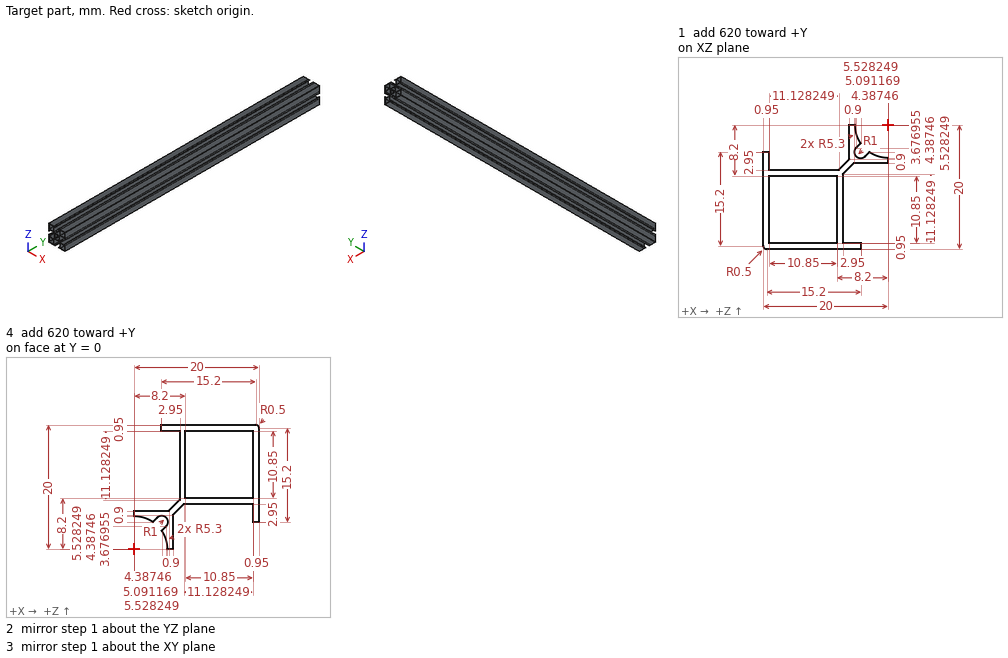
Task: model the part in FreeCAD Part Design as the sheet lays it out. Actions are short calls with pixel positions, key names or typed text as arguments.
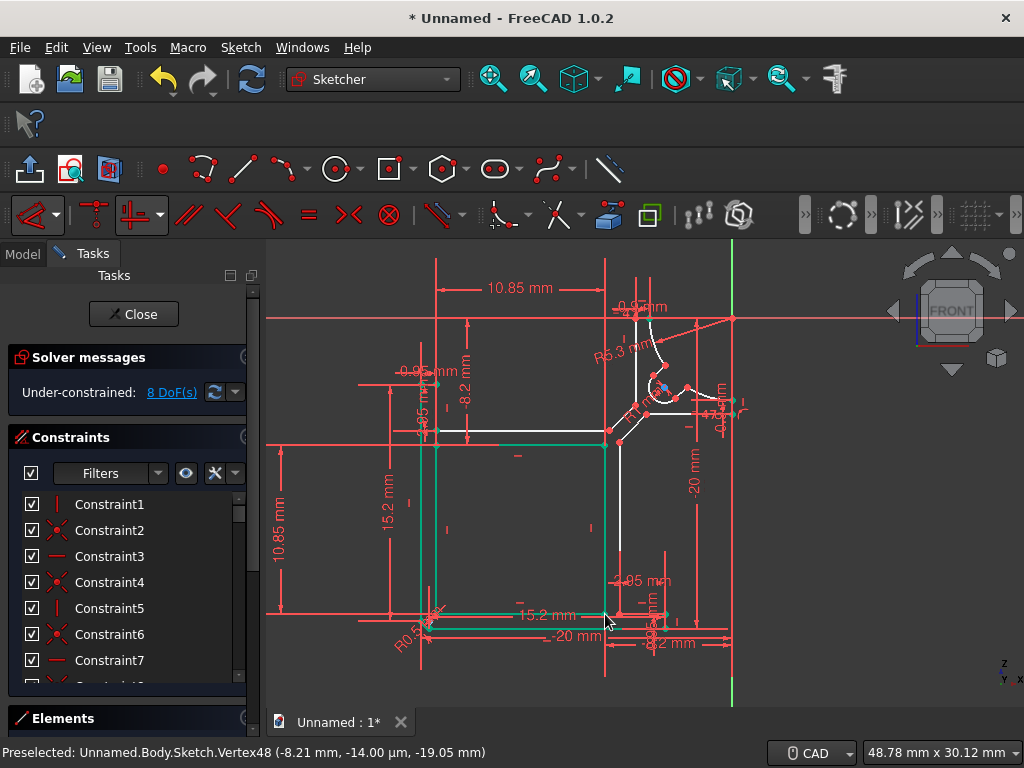
click(636, 379)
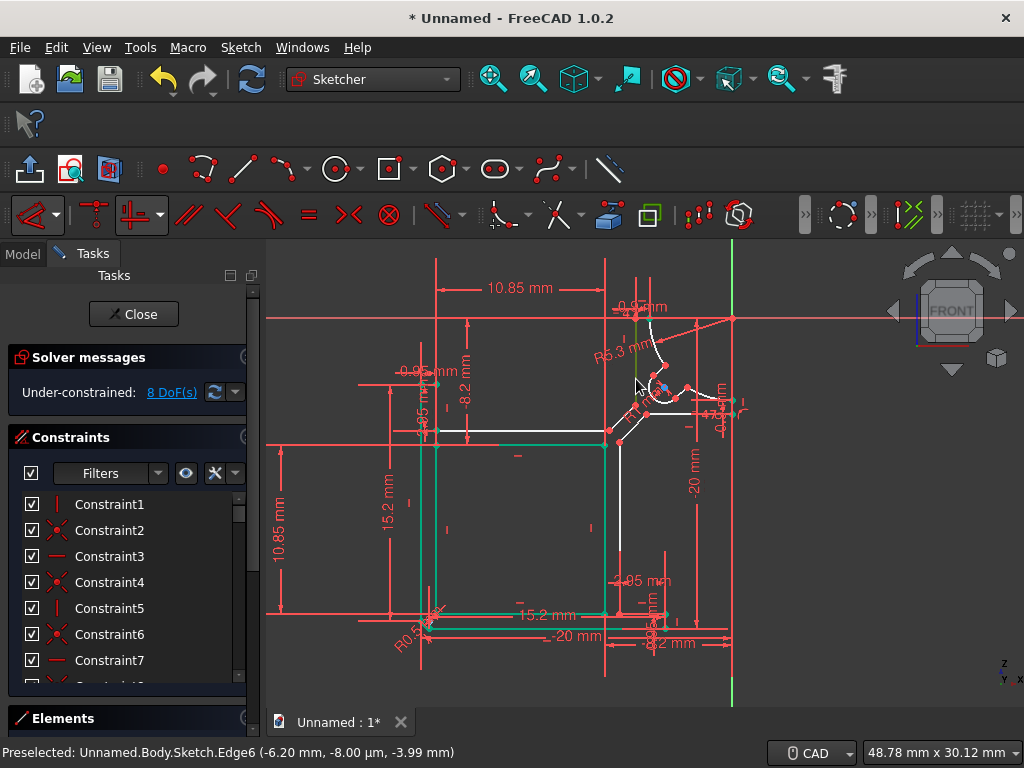
click(58, 216)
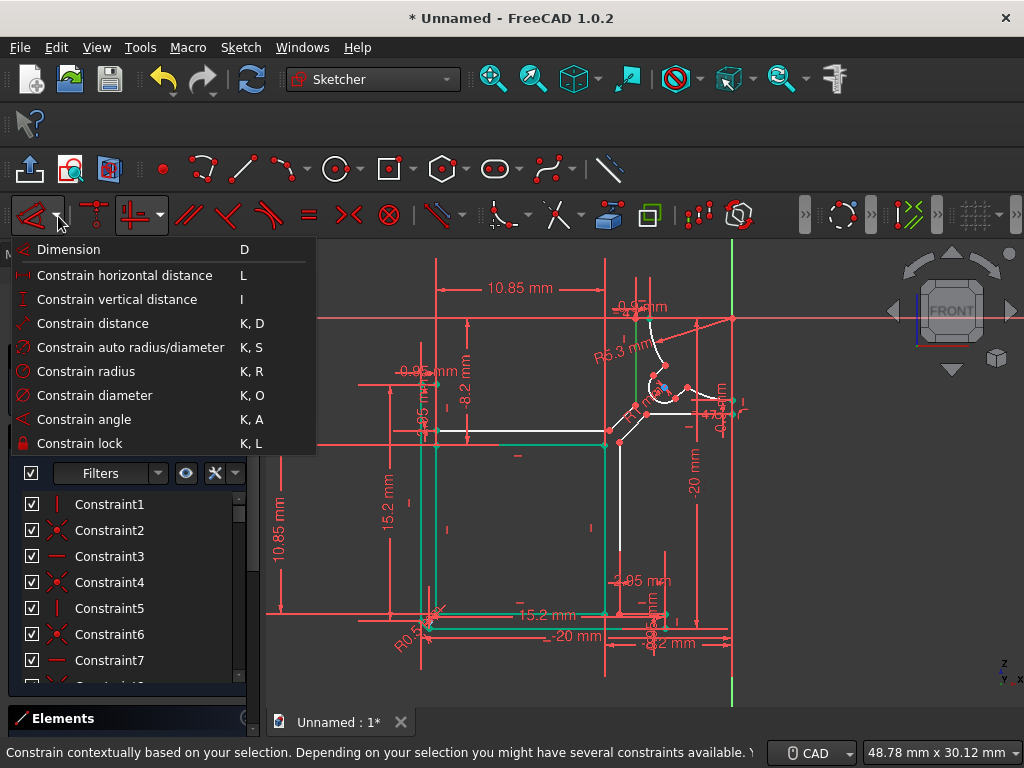
click(164, 299)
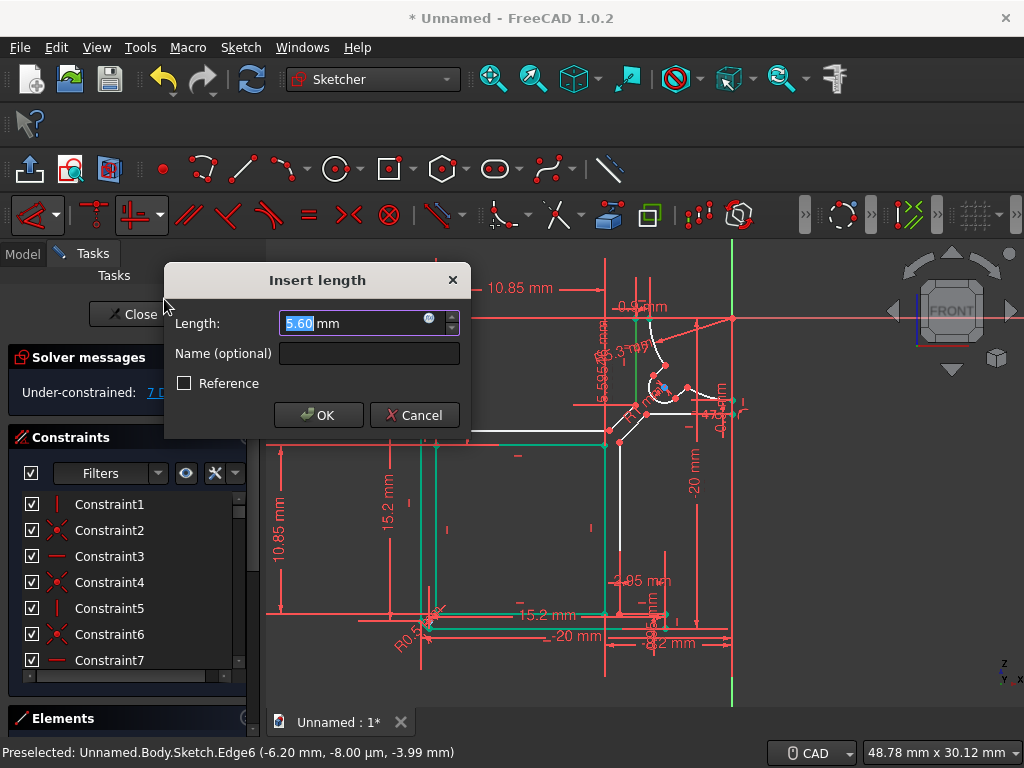
text(5.528249)
key(Return)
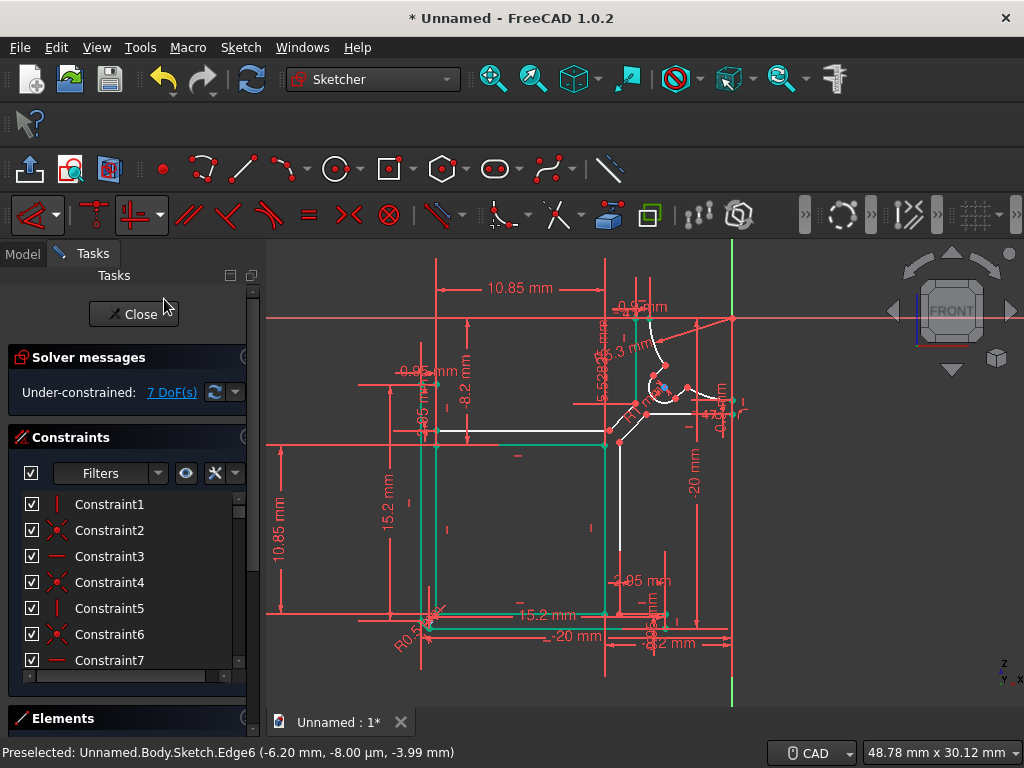
click(672, 414)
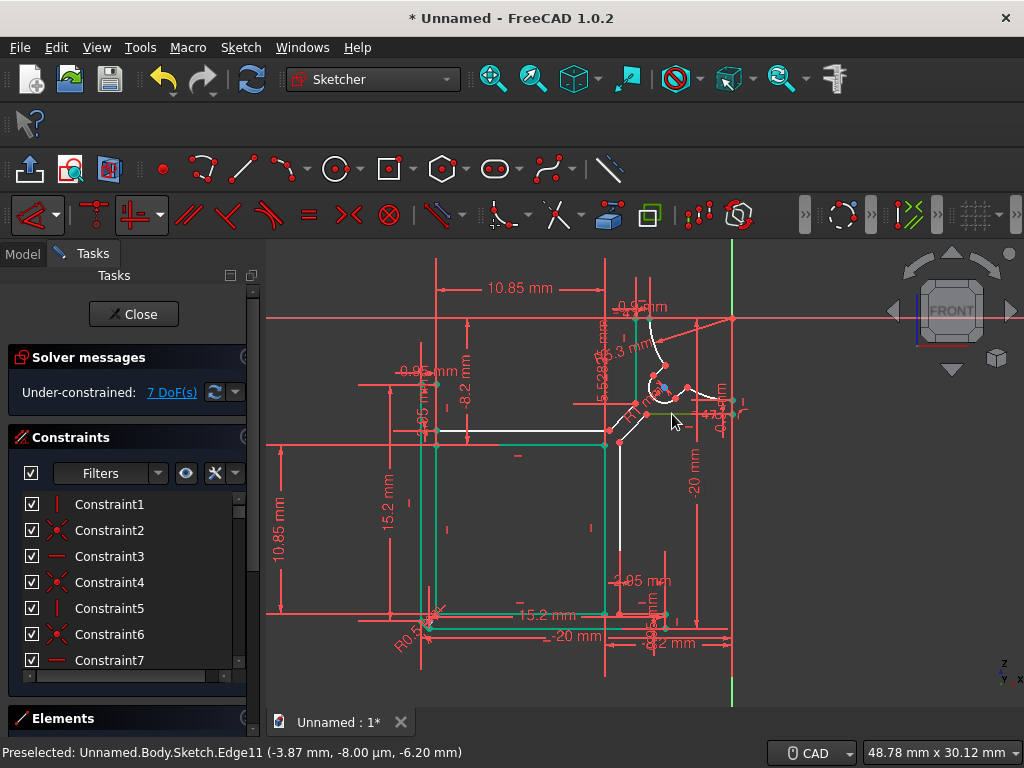
key(l)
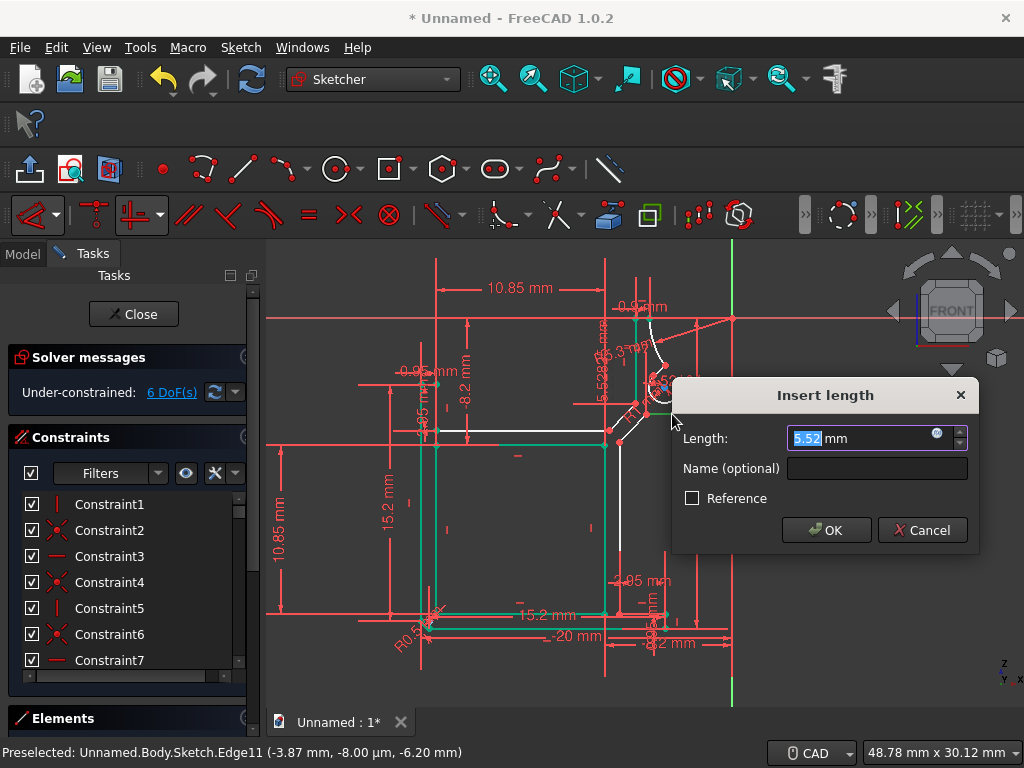
text(5.528249)
key(Return)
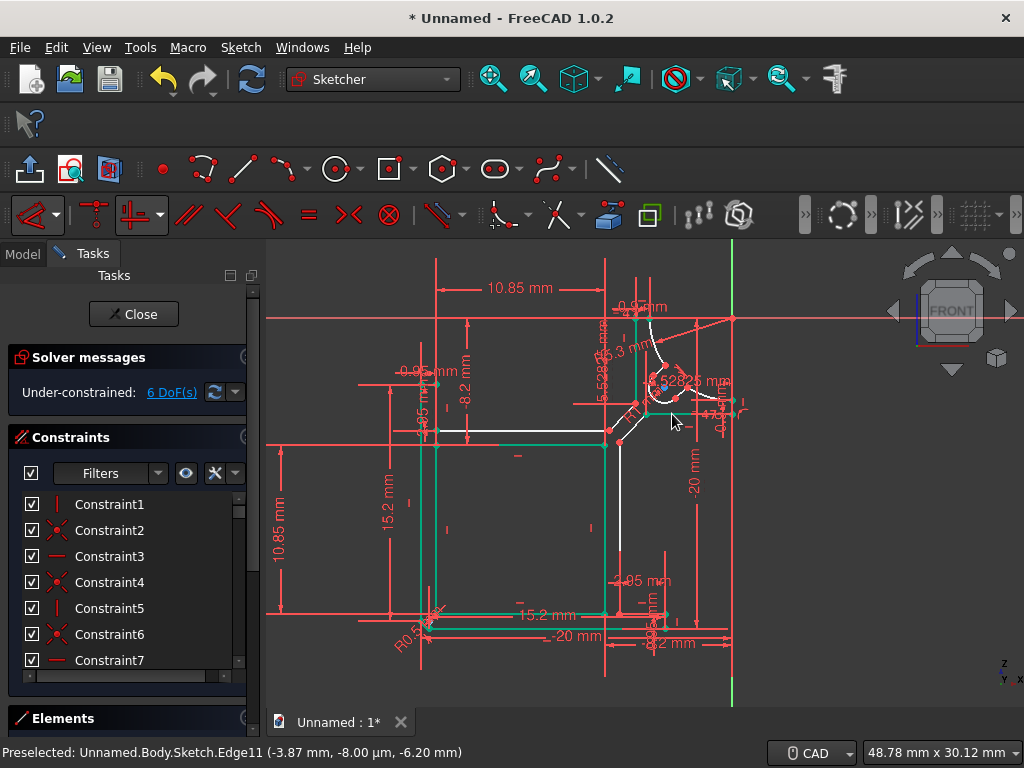
click(665, 366)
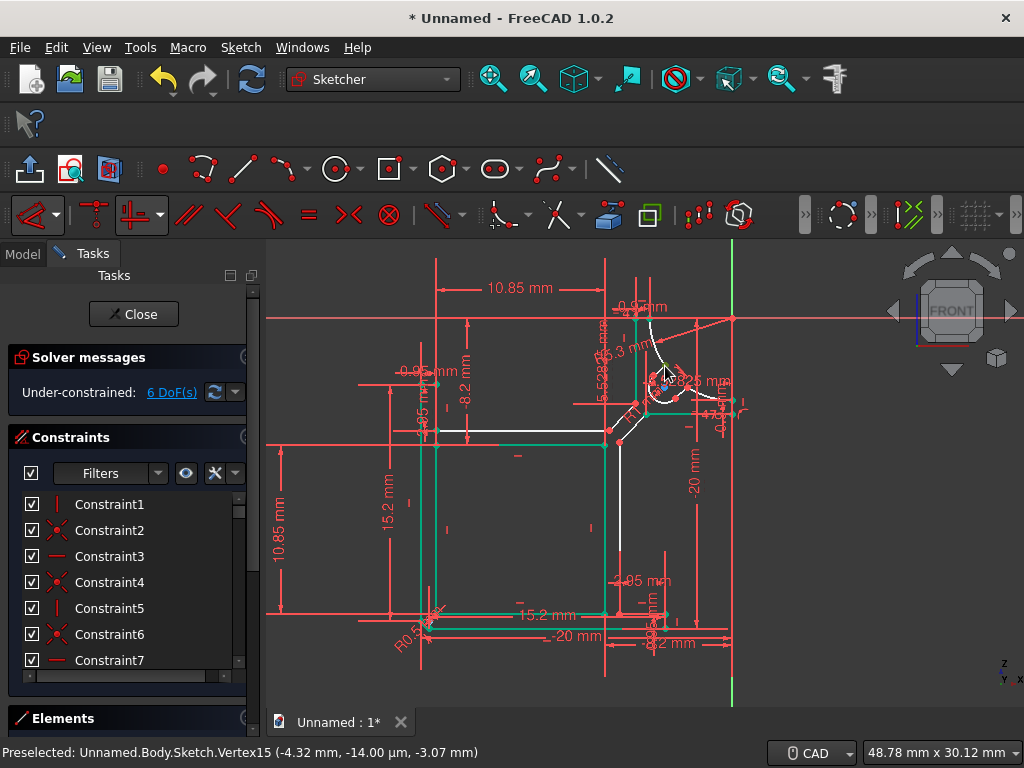
key(l)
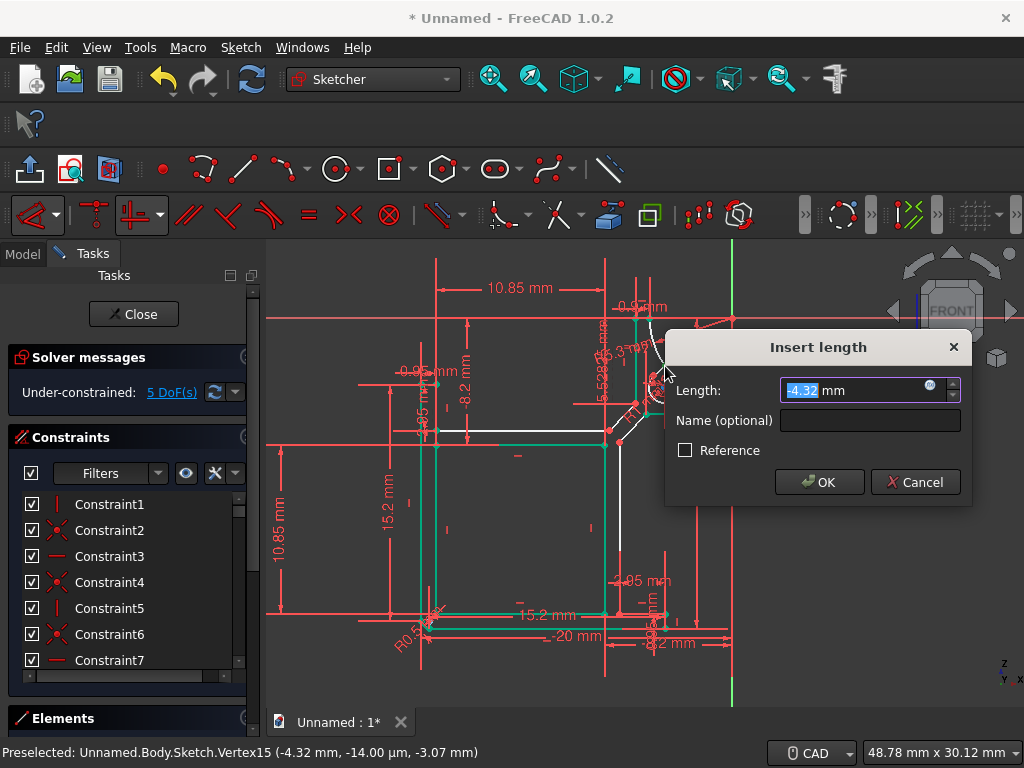
text(-4.38746)
key(Return)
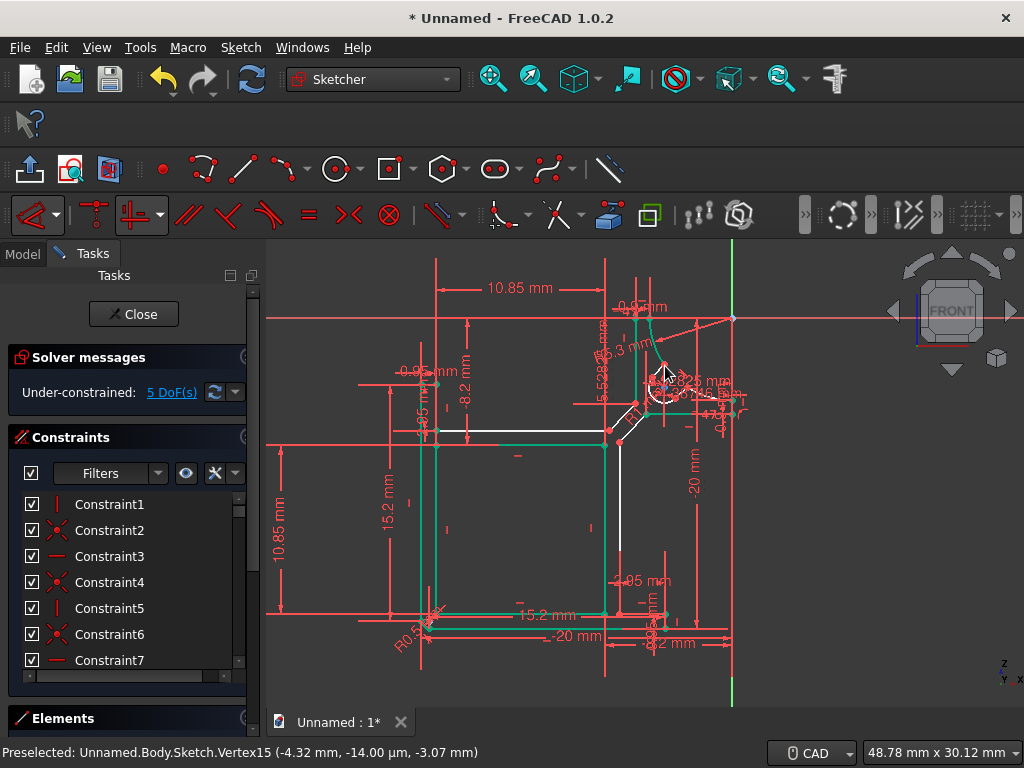
click(687, 387)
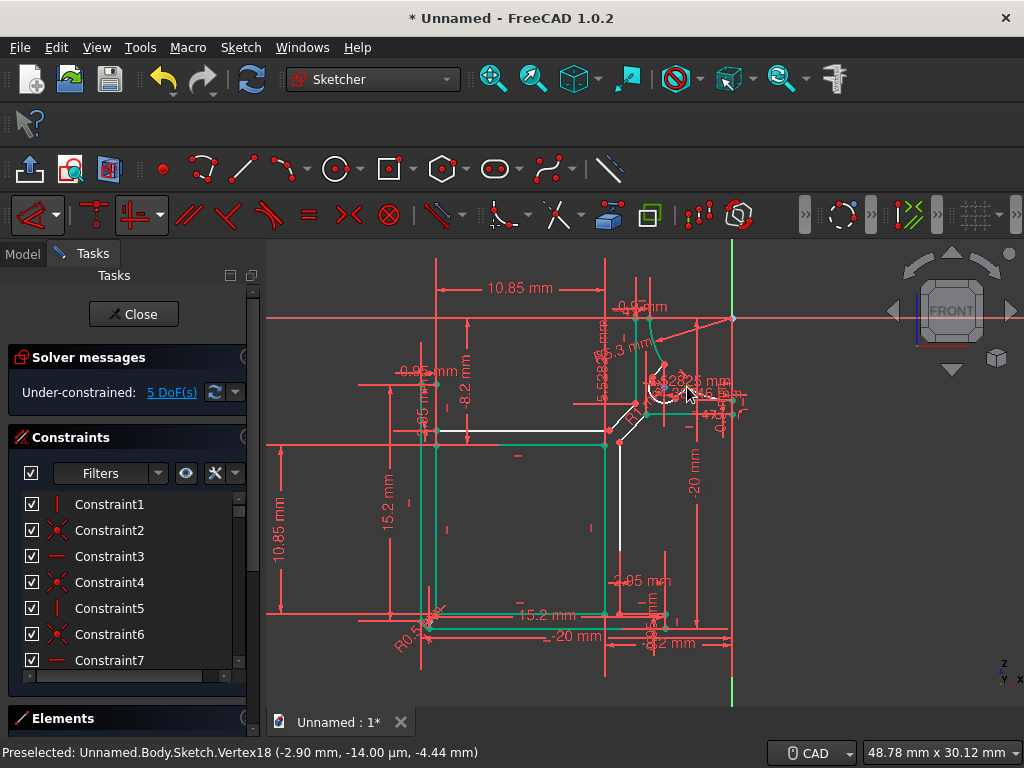
click(58, 216)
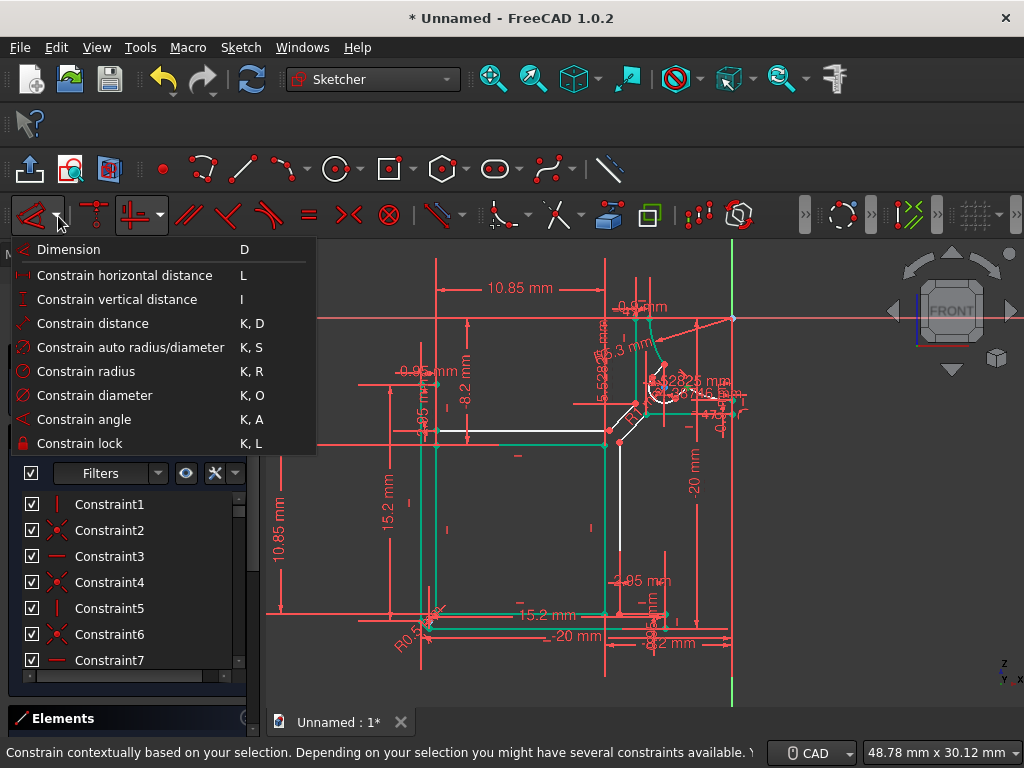
click(164, 299)